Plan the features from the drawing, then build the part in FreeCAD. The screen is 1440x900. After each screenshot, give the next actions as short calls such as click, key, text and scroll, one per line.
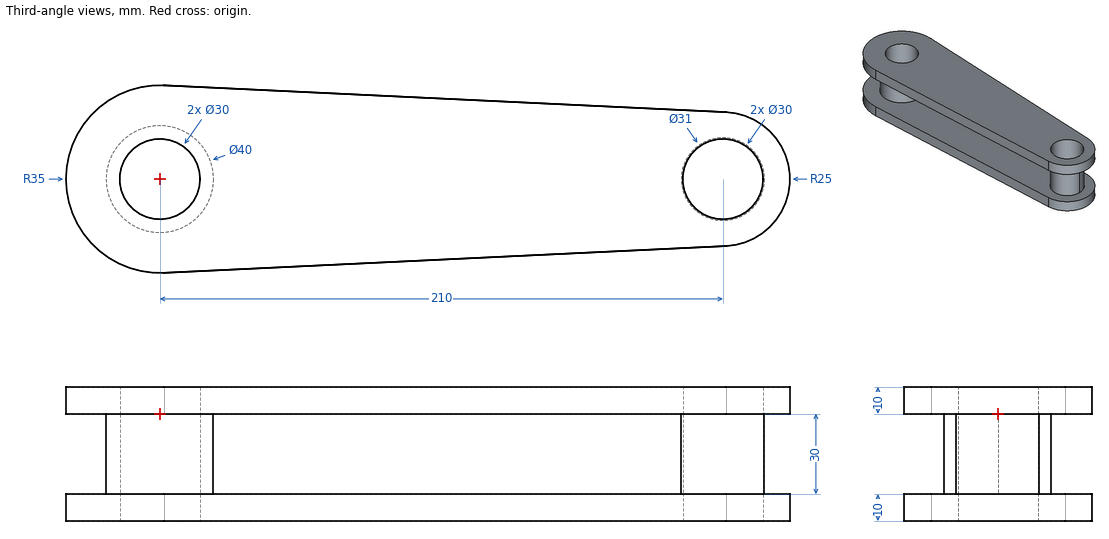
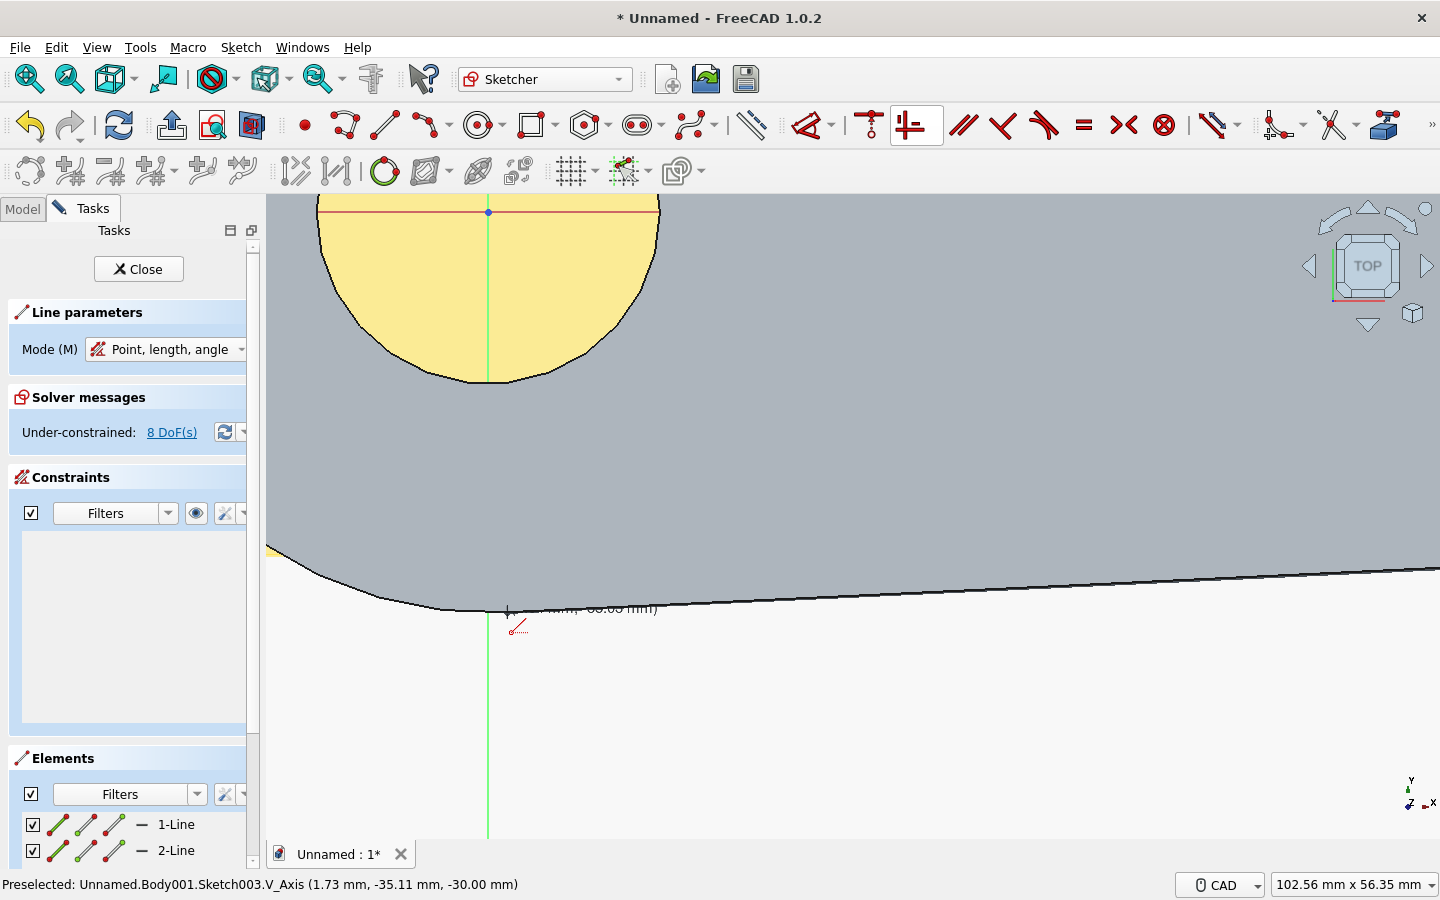
click(426, 126)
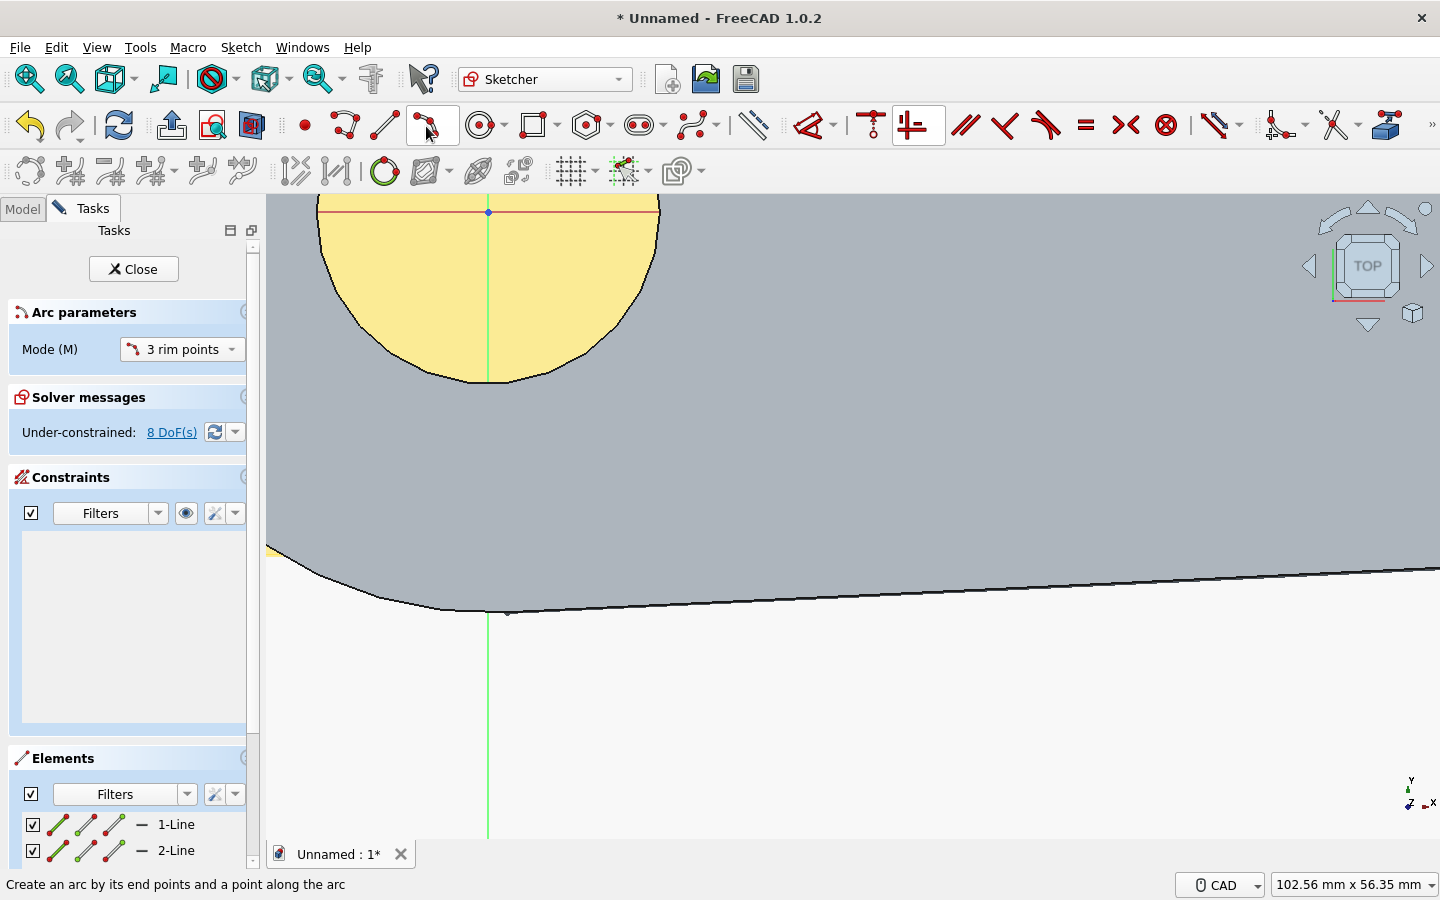
scroll(507, 616, down, 7)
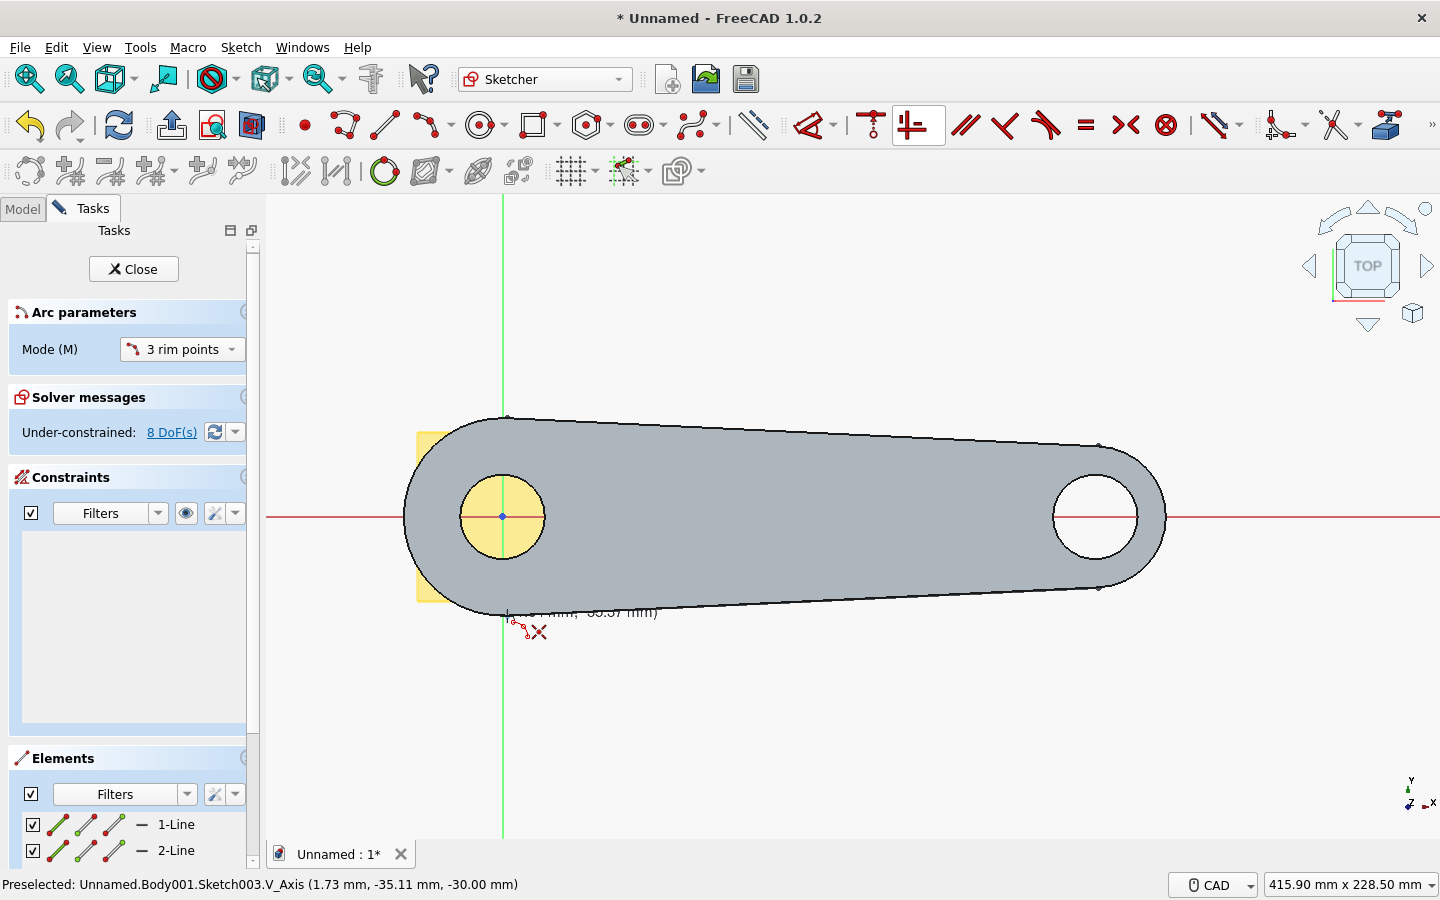
click(1099, 447)
click(1099, 588)
click(1163, 538)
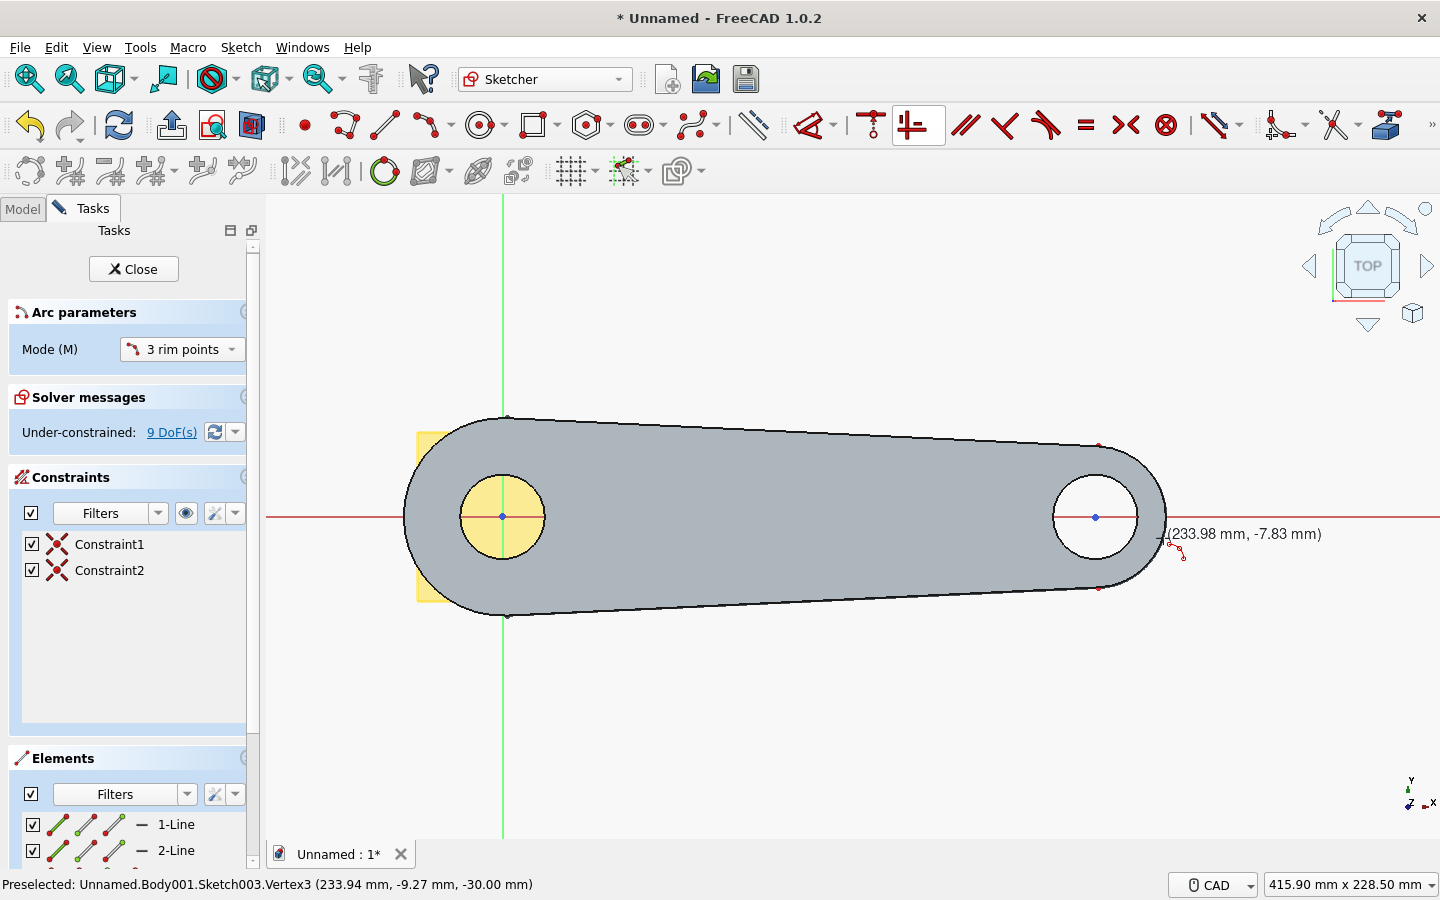
scroll(507, 616, up, 7)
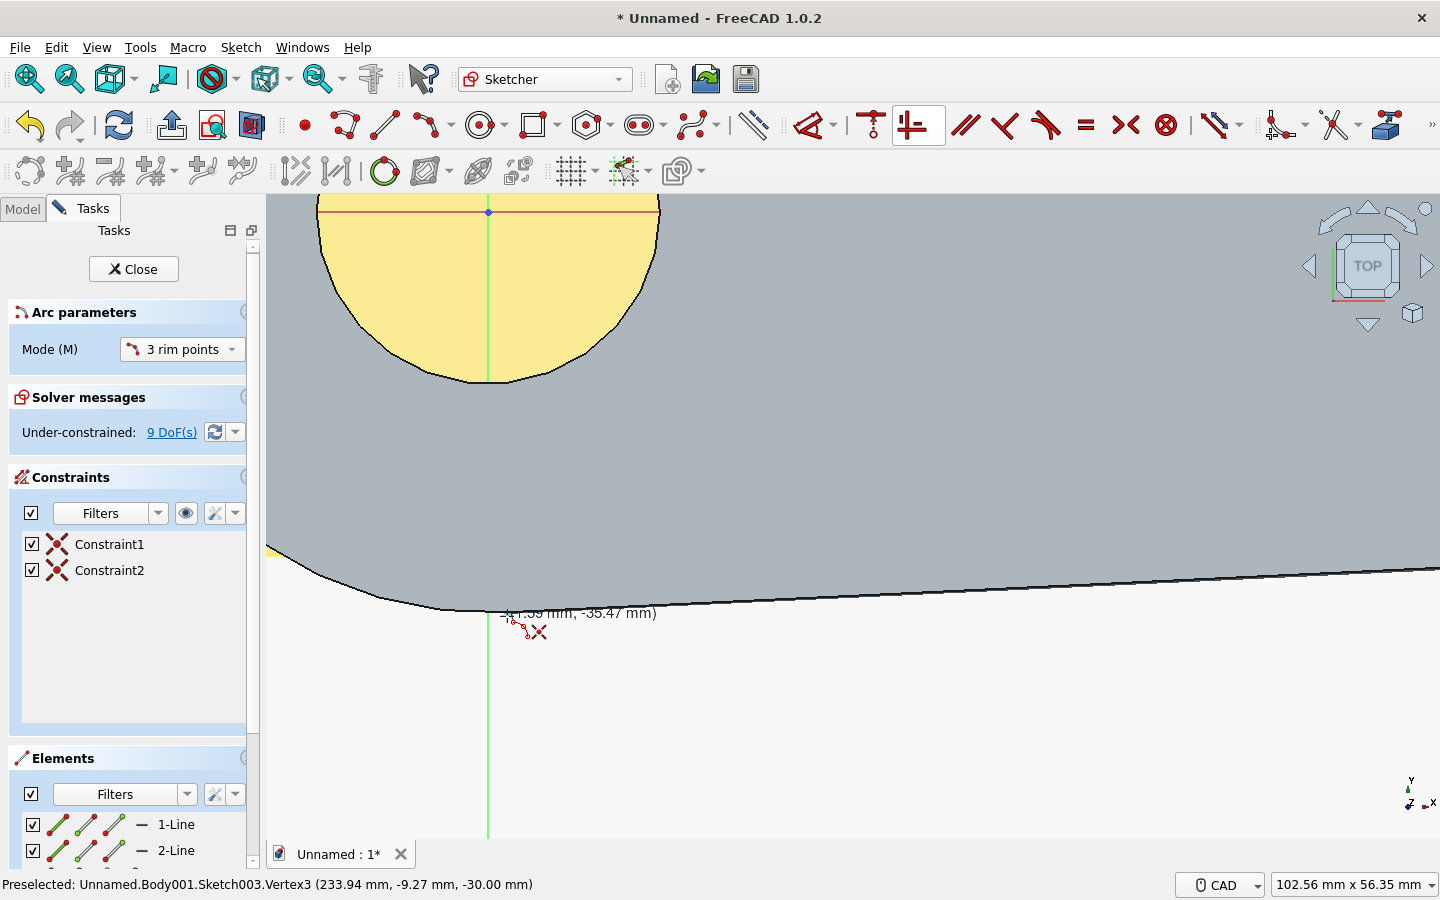
click(507, 613)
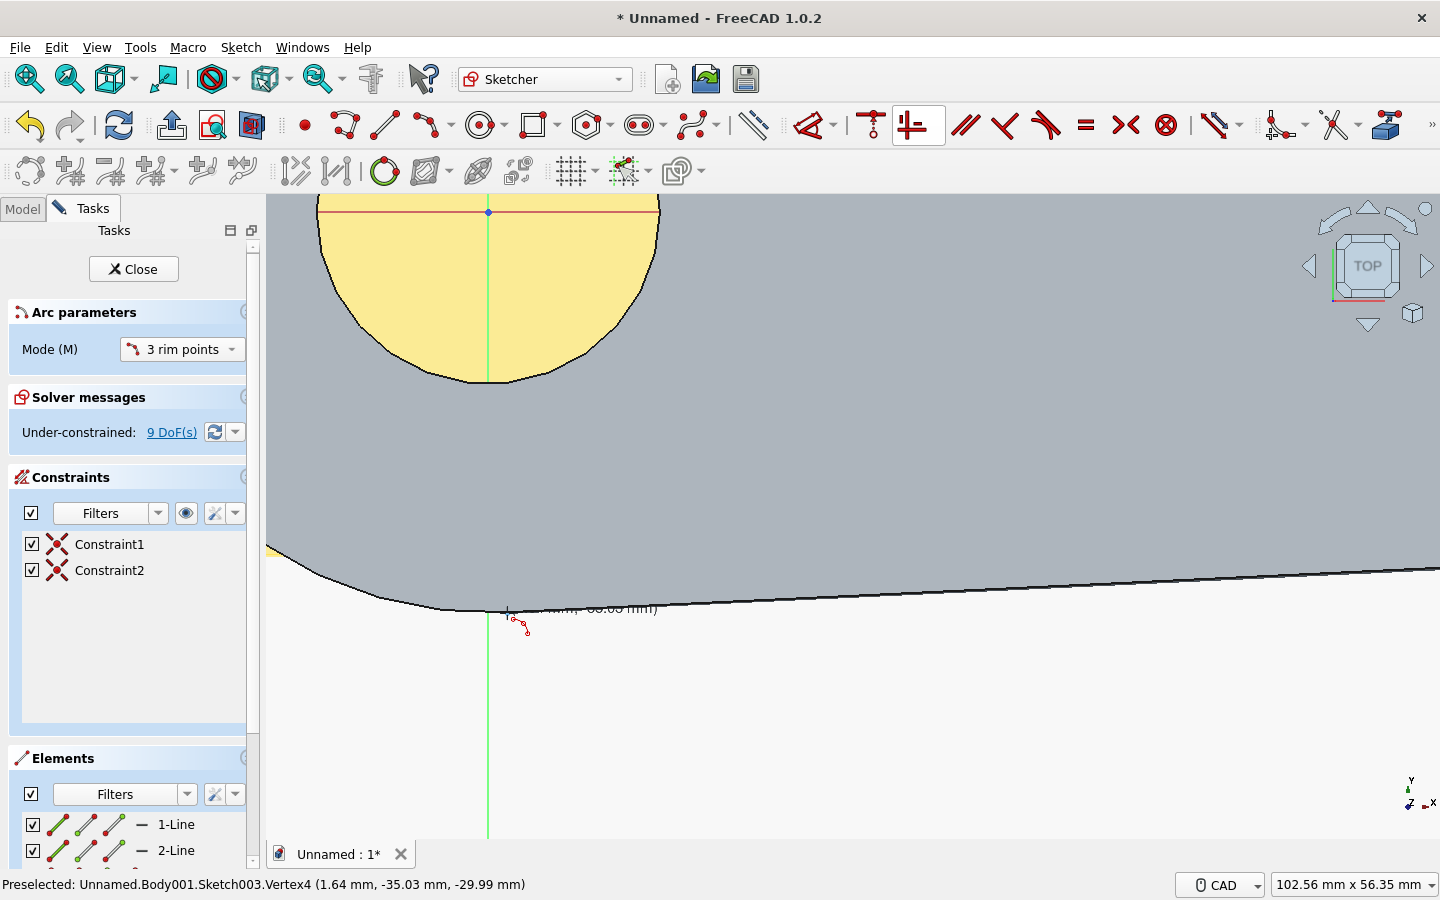
scroll(507, 616, down, 7)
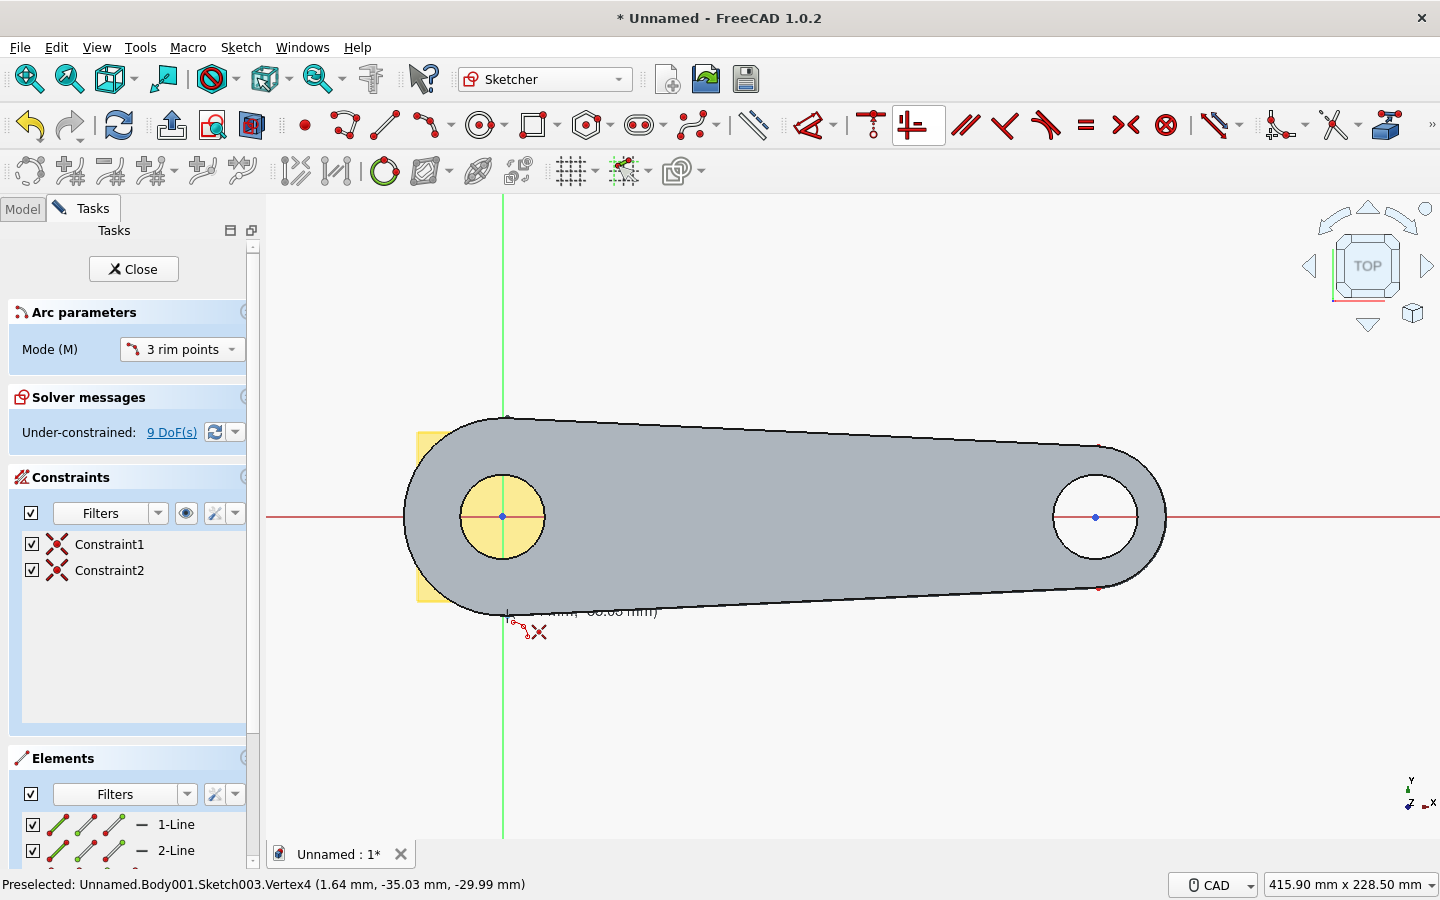
scroll(507, 418, up, 7)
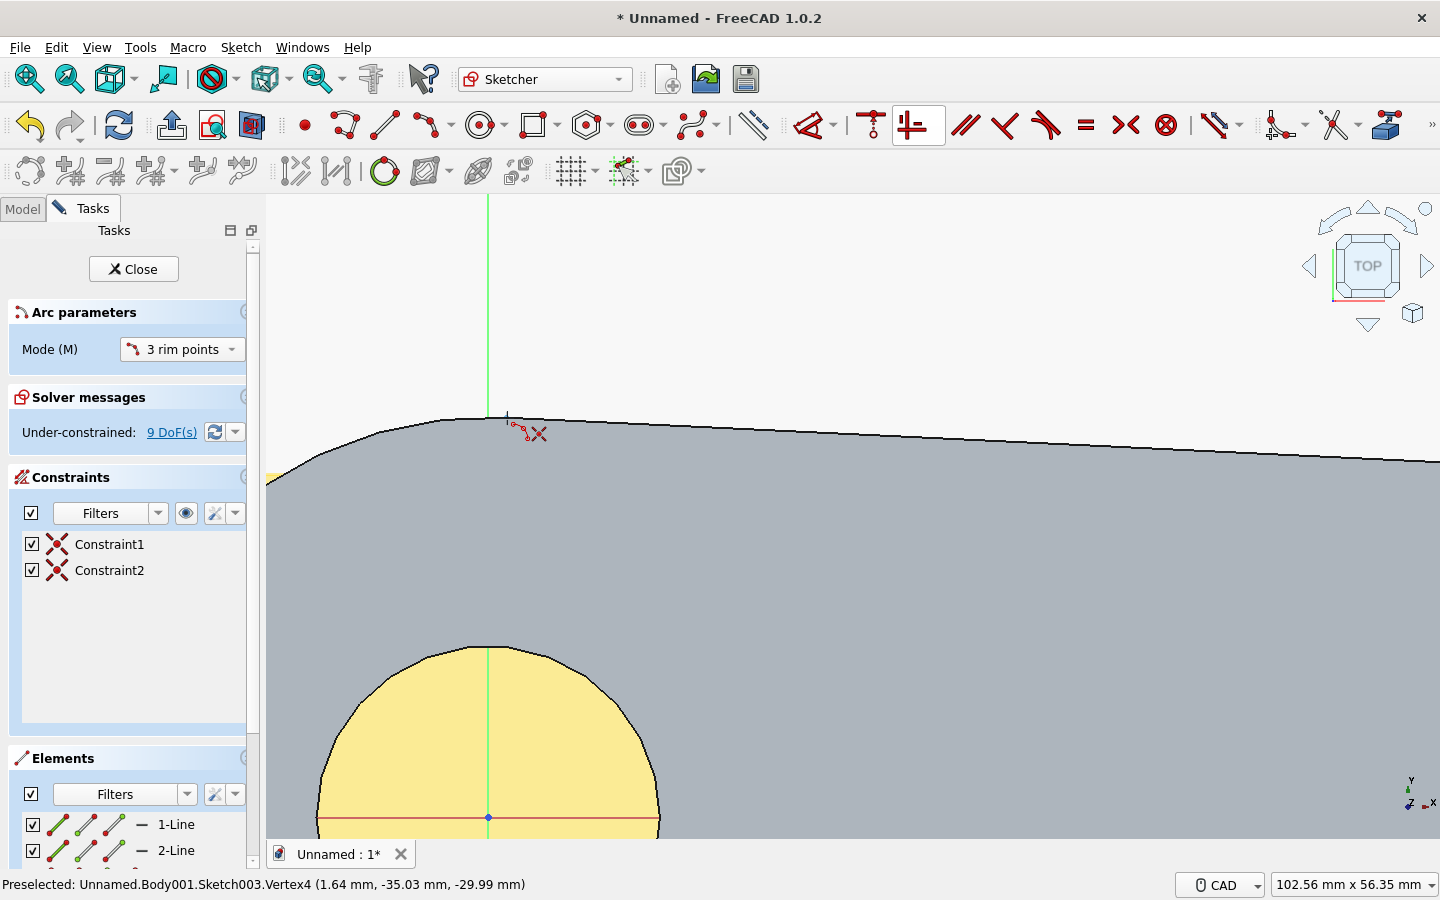
click(507, 419)